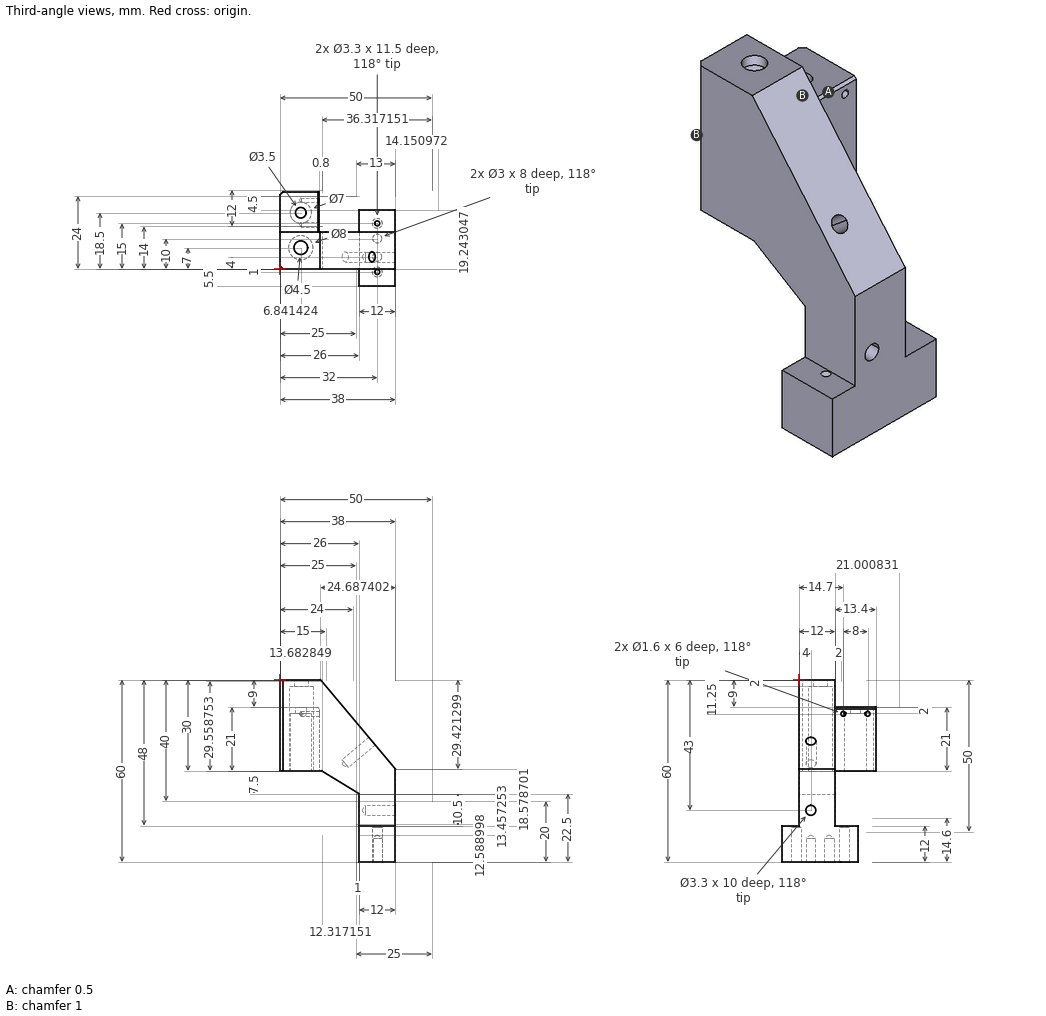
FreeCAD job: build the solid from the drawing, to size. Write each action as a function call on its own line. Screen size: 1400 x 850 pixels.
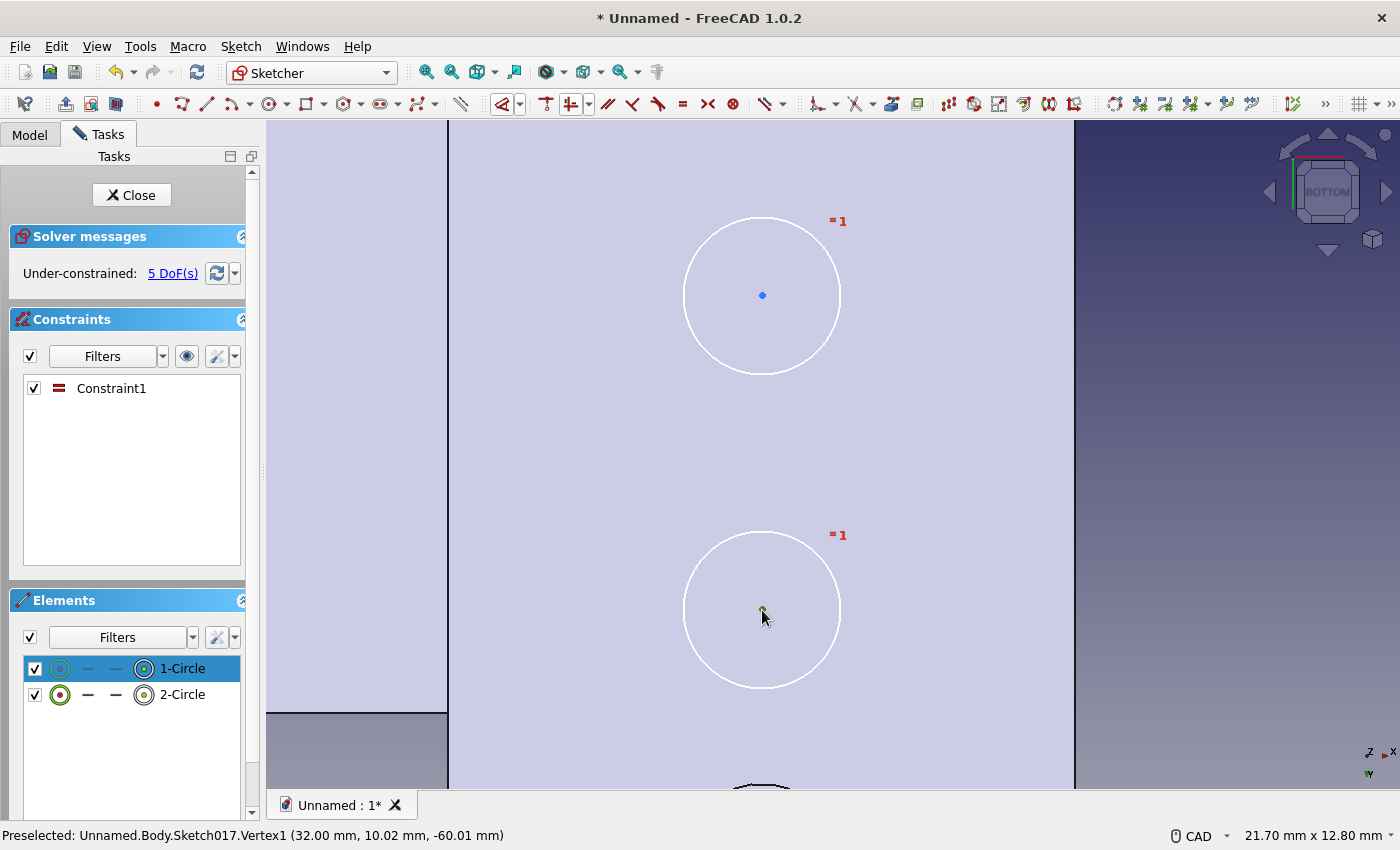
click(762, 296)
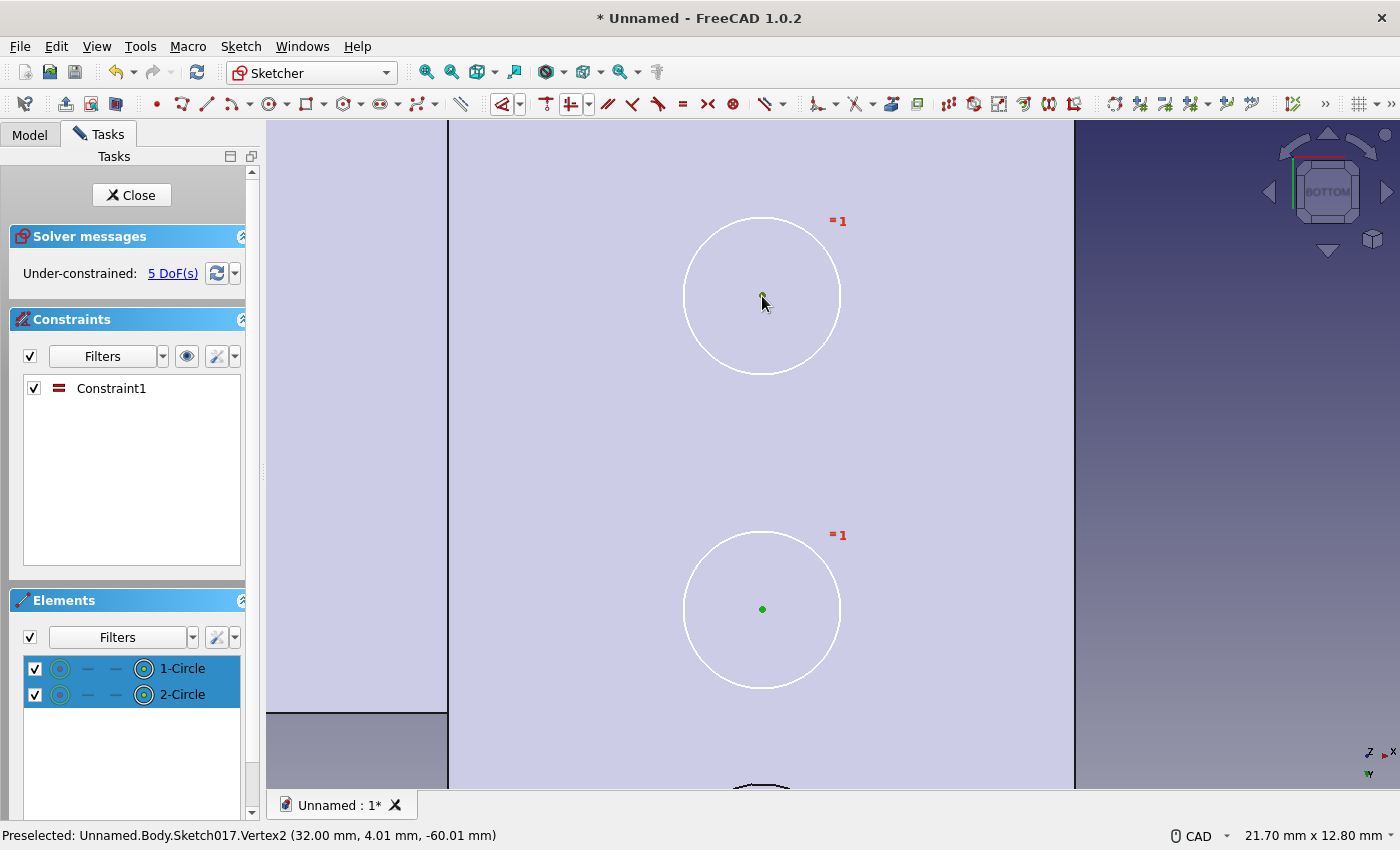
click(588, 104)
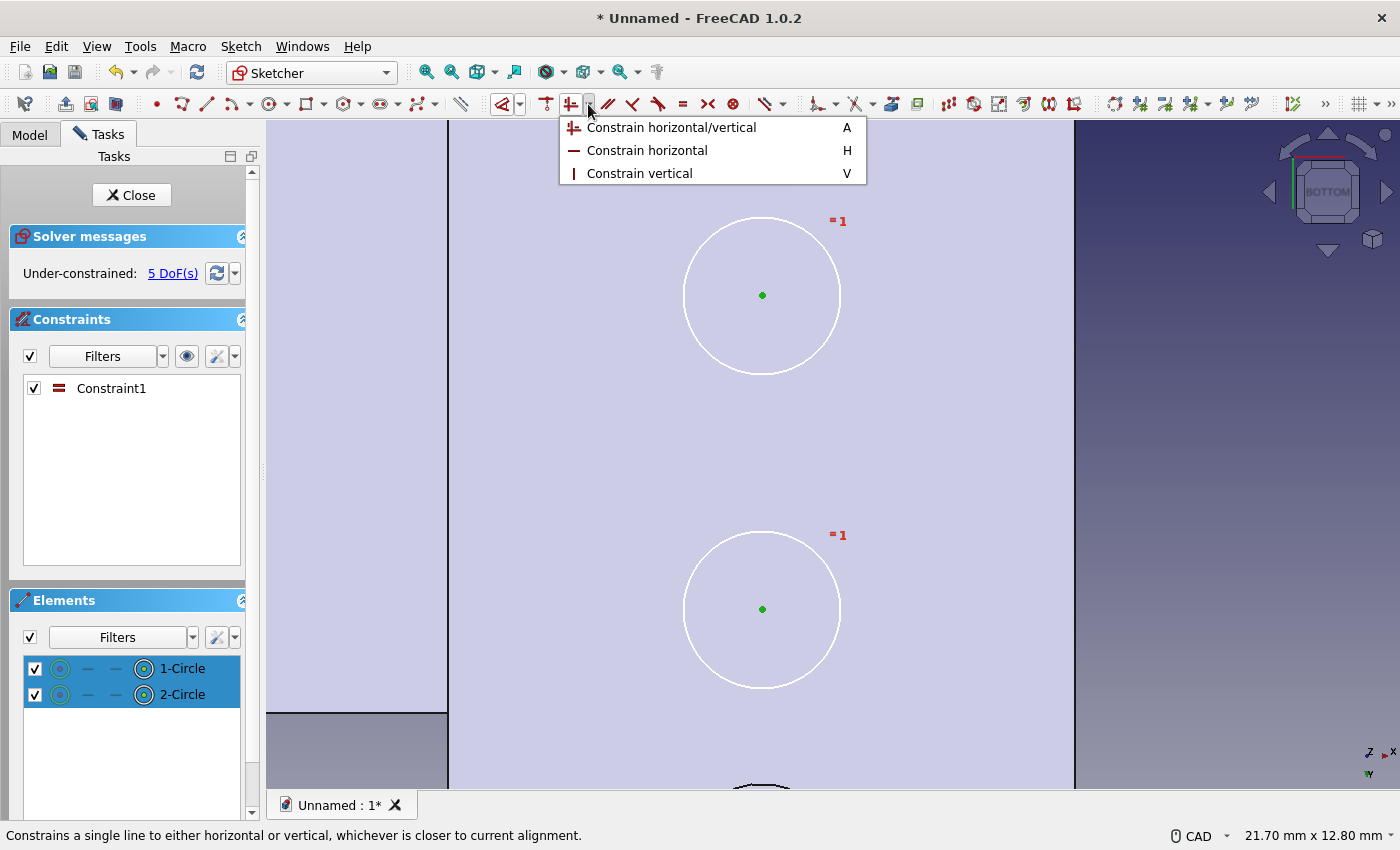
click(713, 174)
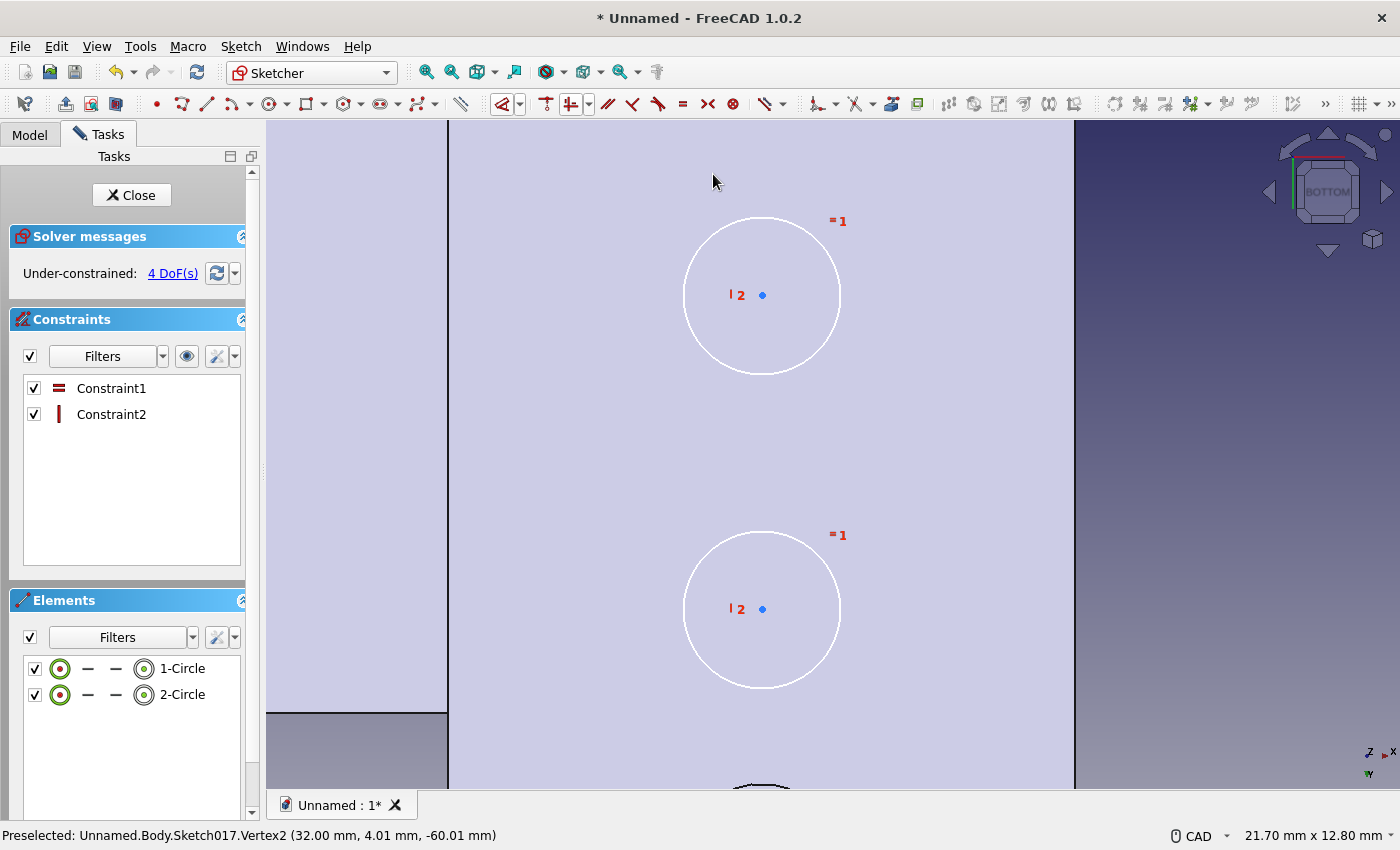
click(817, 554)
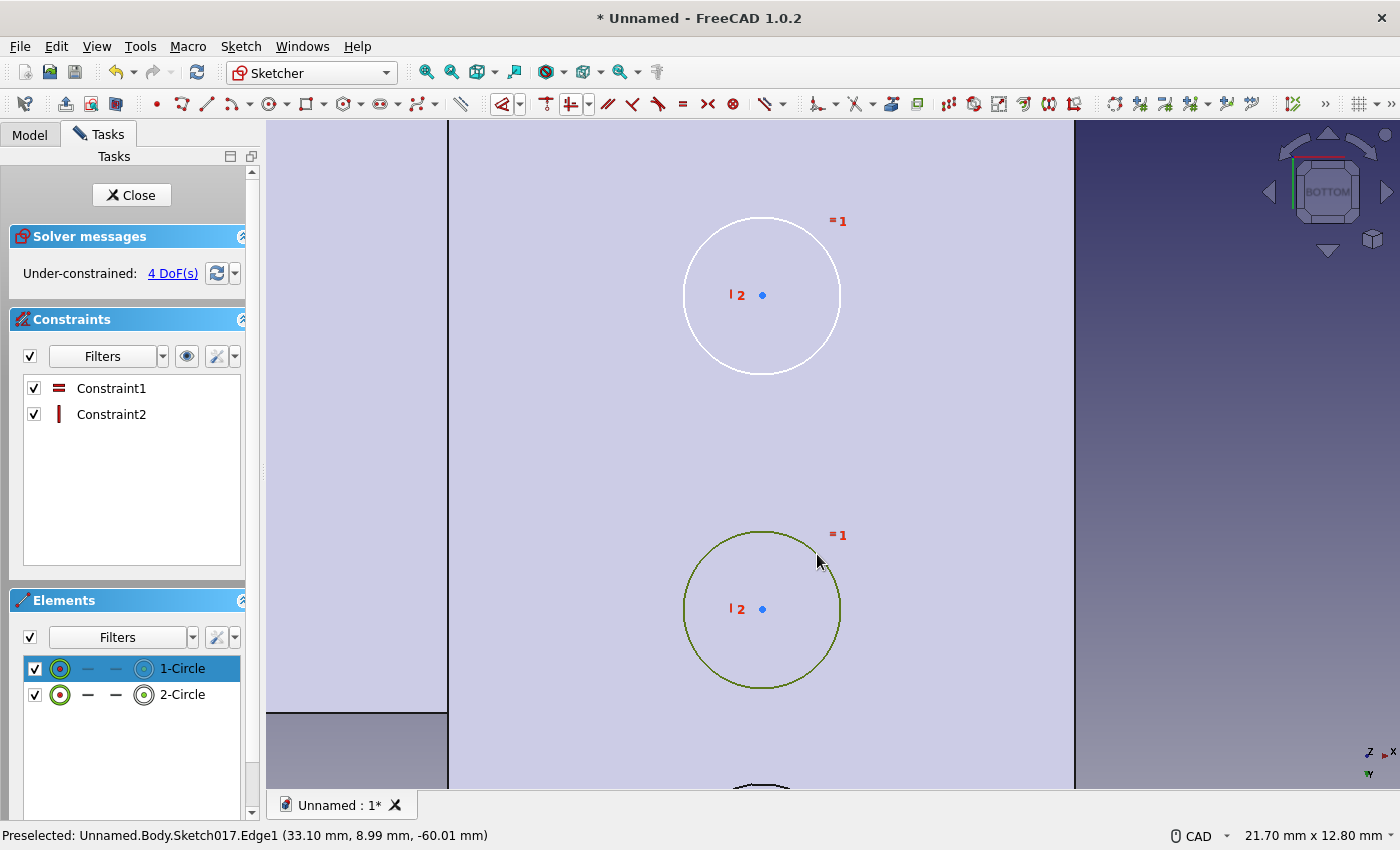
click(520, 104)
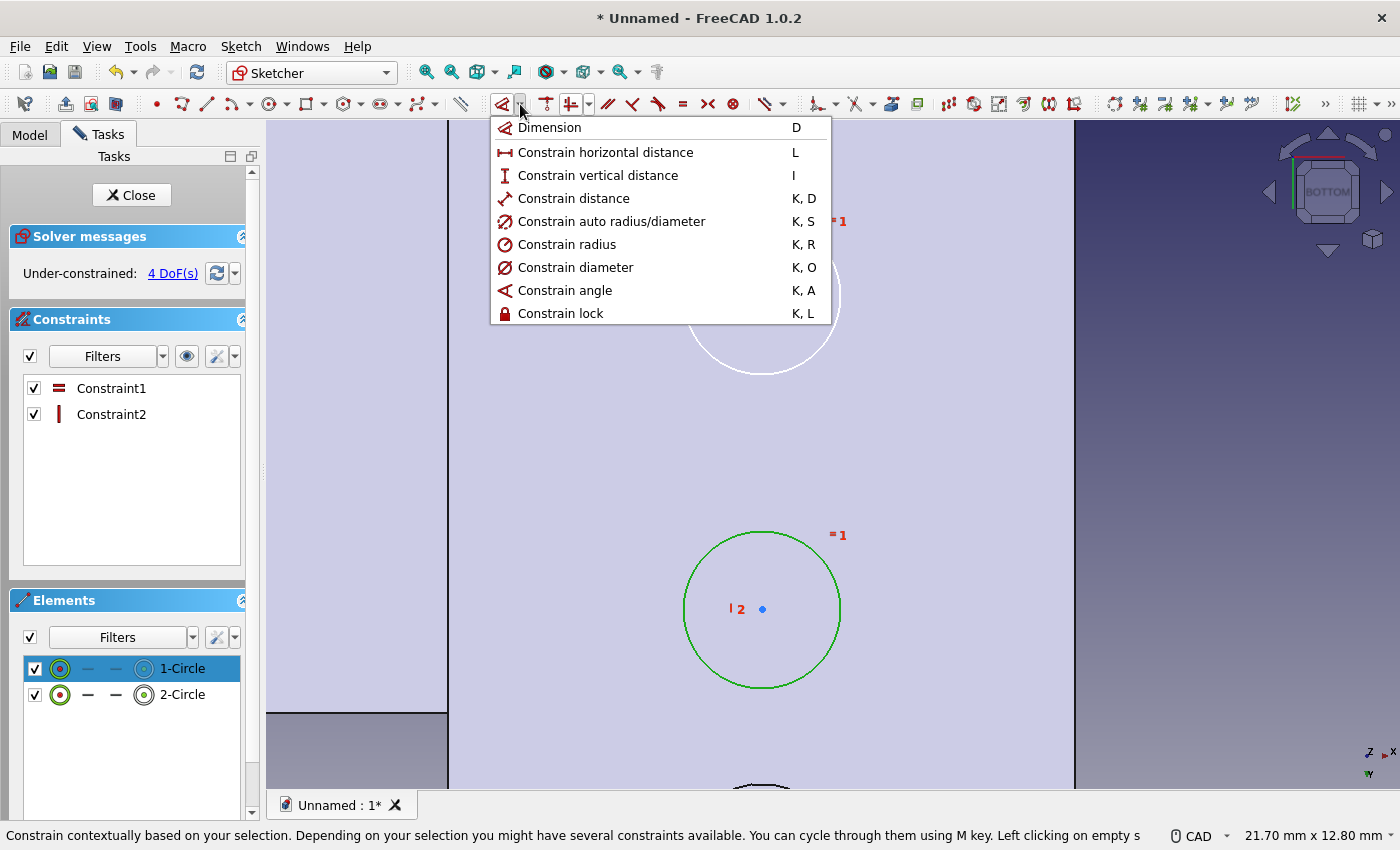
click(661, 268)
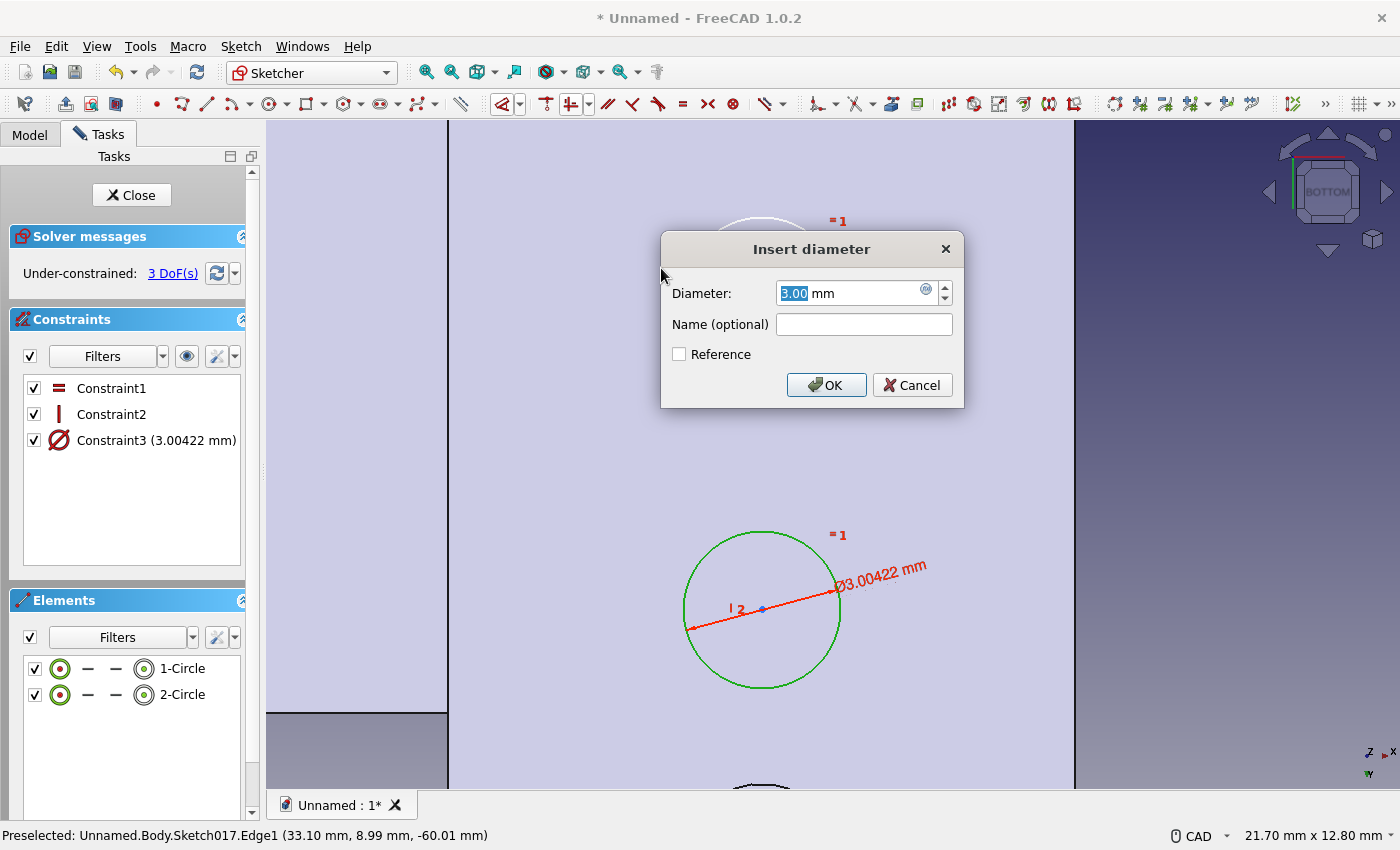
text(3)
key(Return)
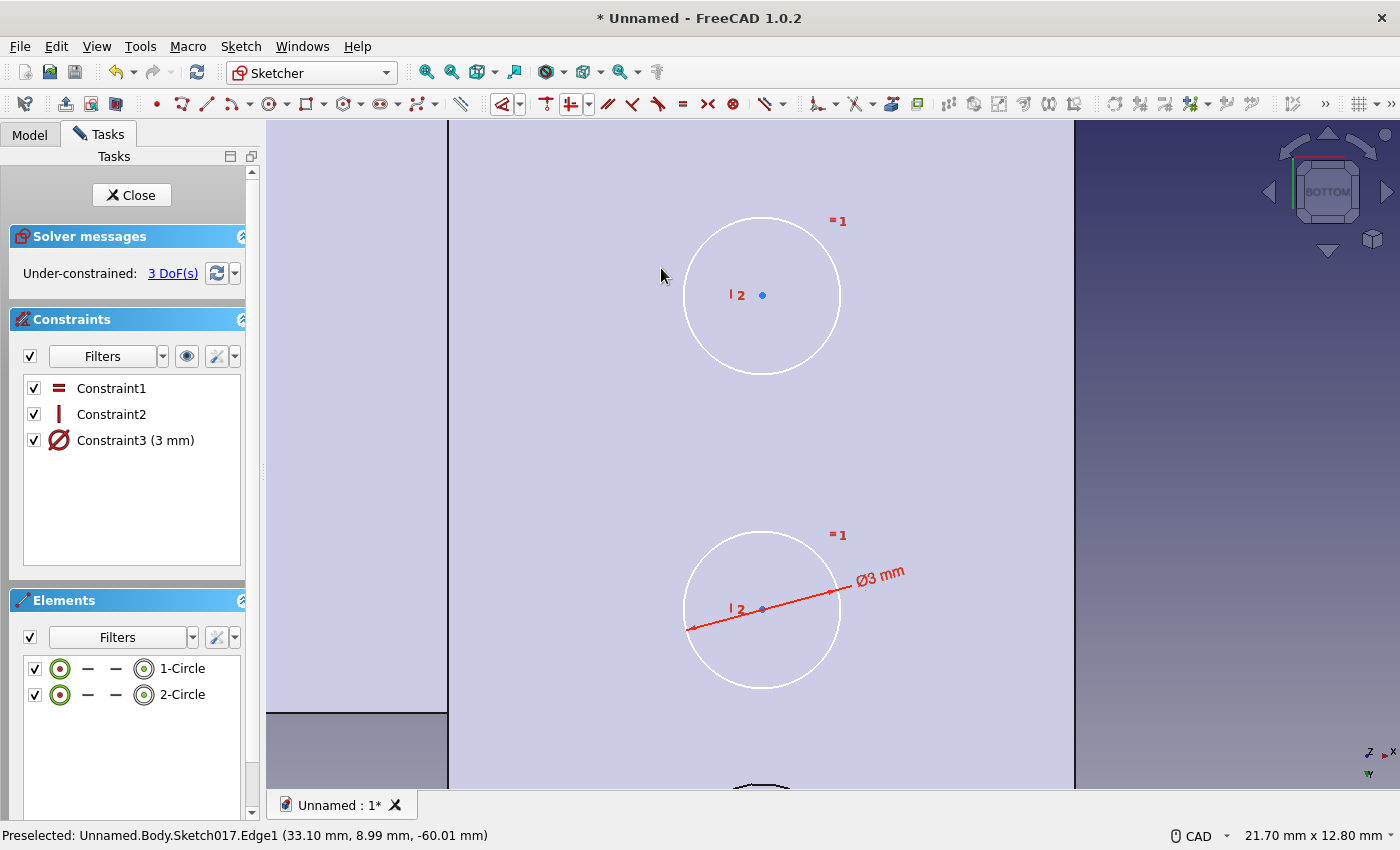
click(762, 296)